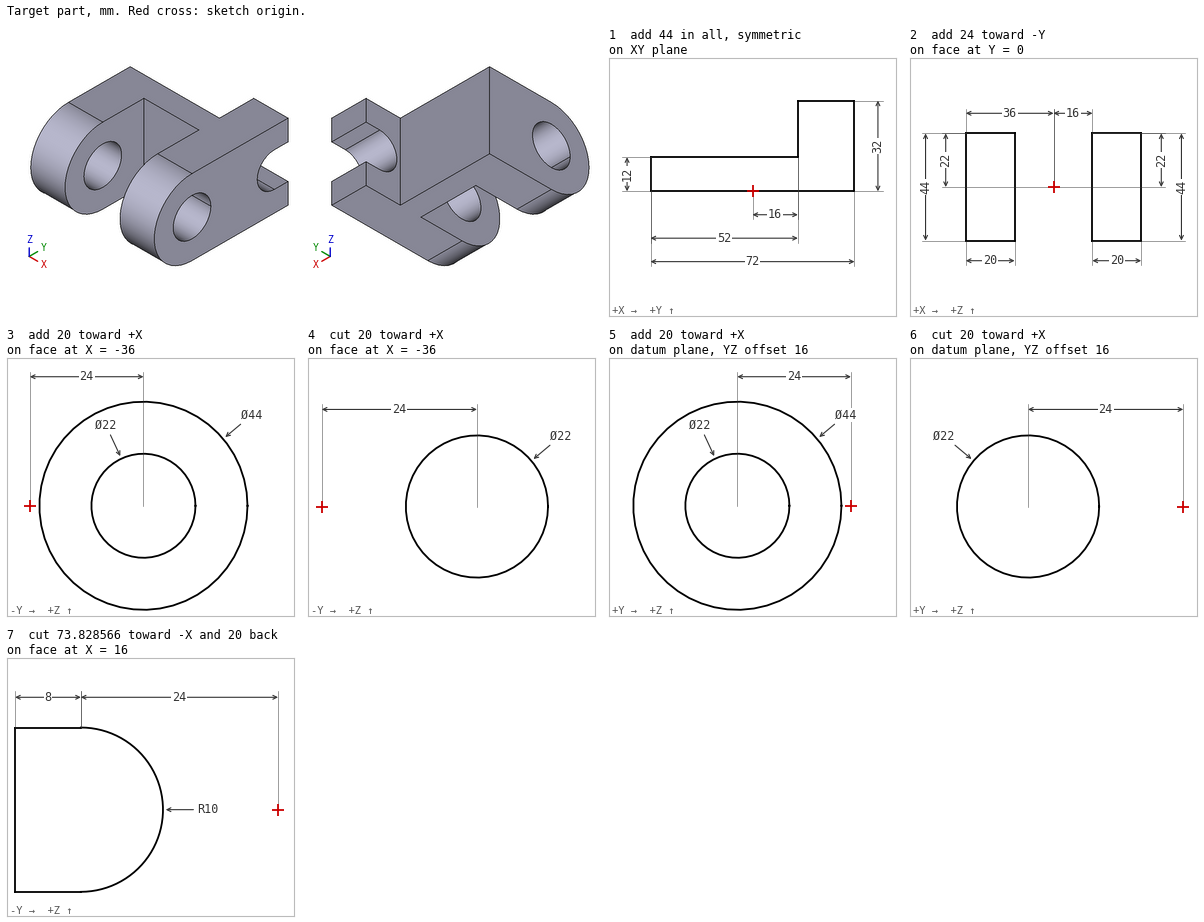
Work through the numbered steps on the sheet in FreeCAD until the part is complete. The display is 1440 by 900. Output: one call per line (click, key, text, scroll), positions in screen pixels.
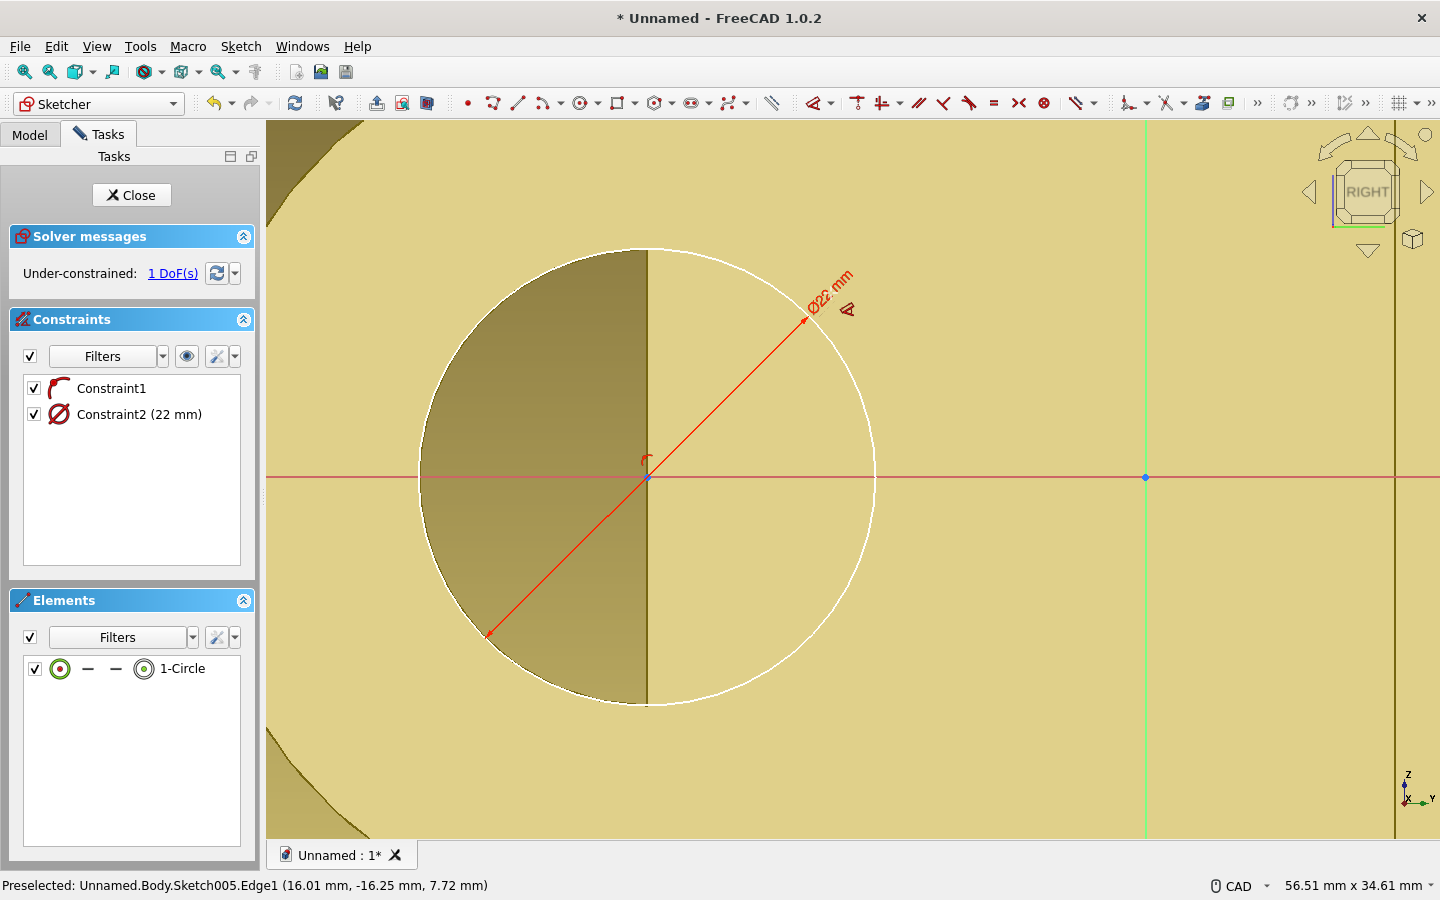
click(647, 477)
click(896, 511)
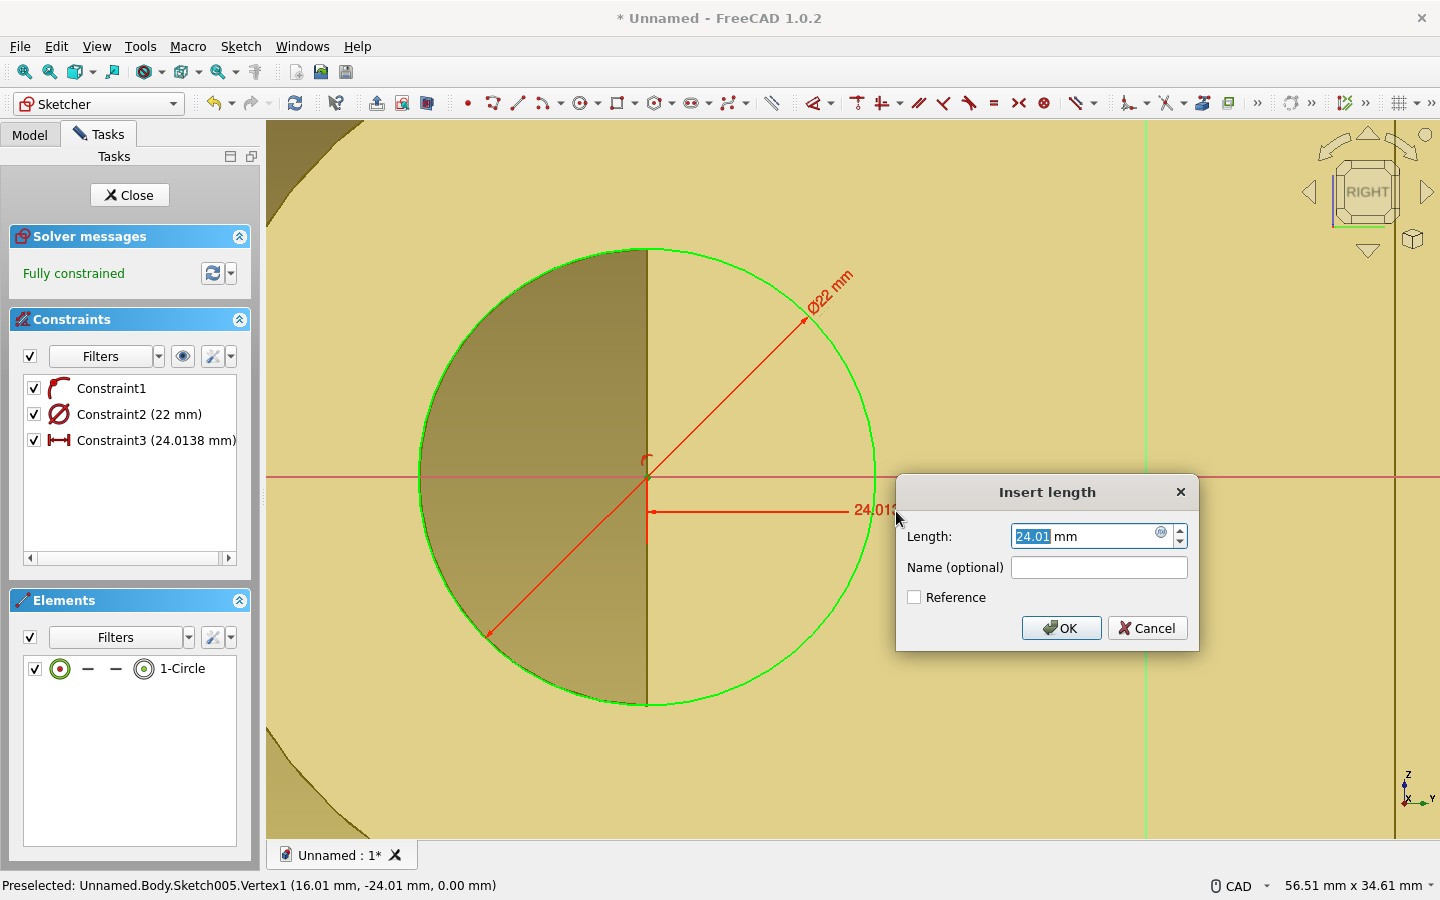
text(24)
key(Return)
key(Escape)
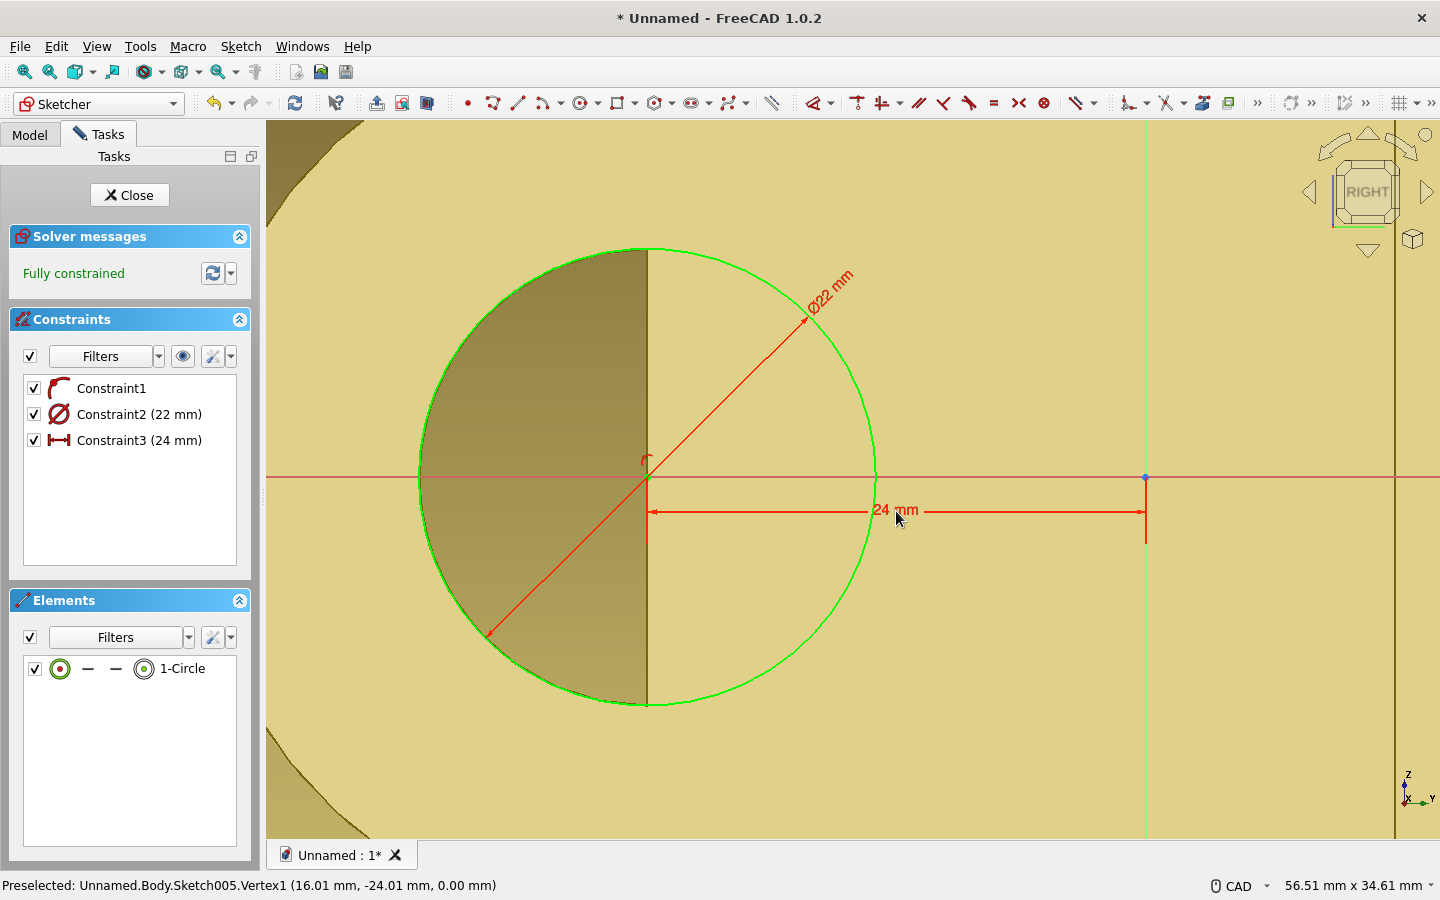
click(130, 195)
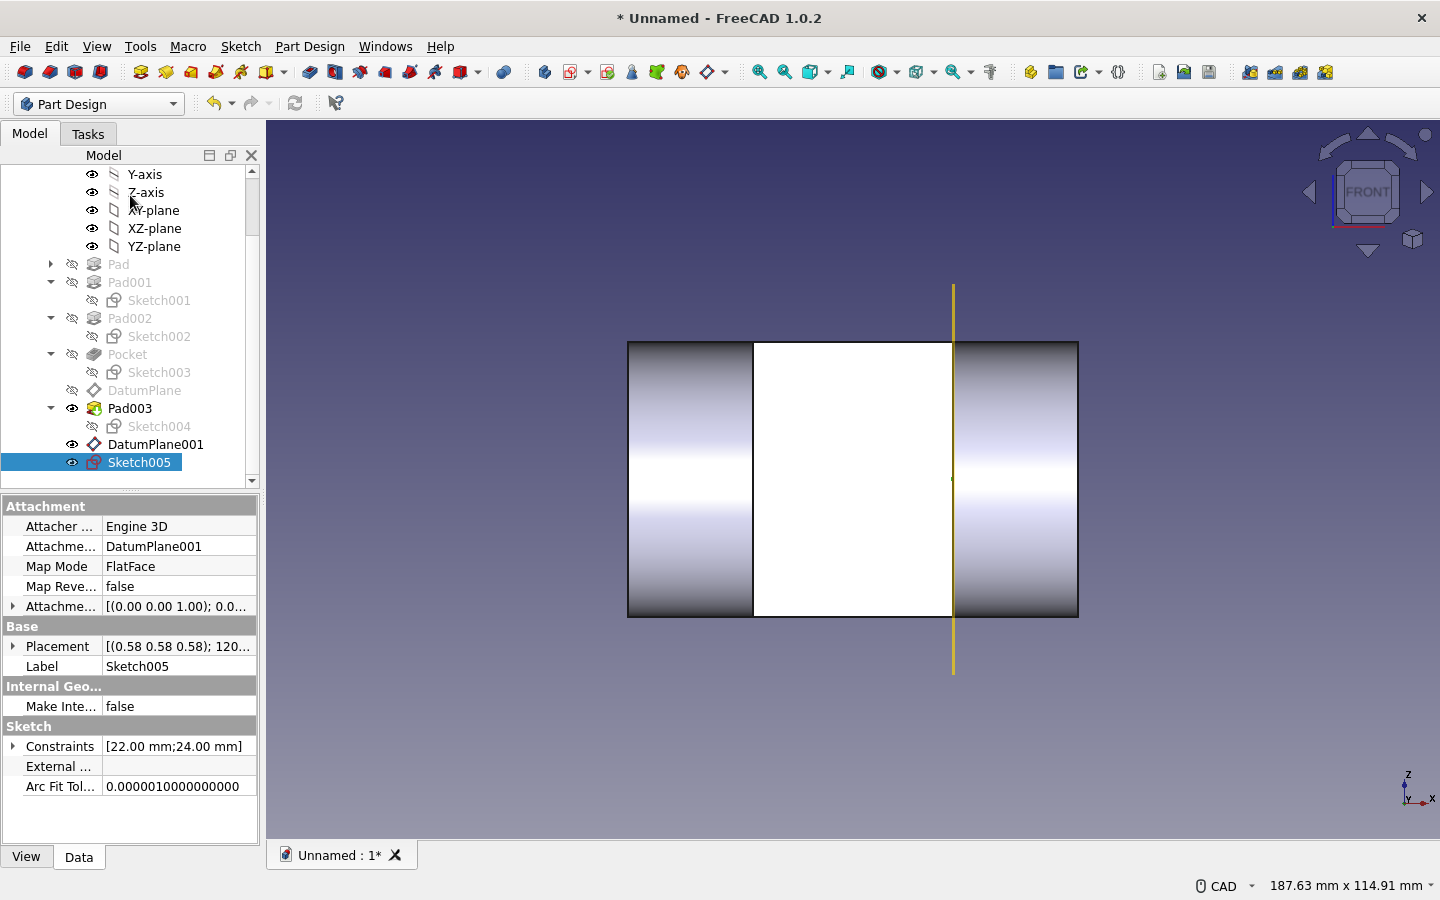
click(310, 72)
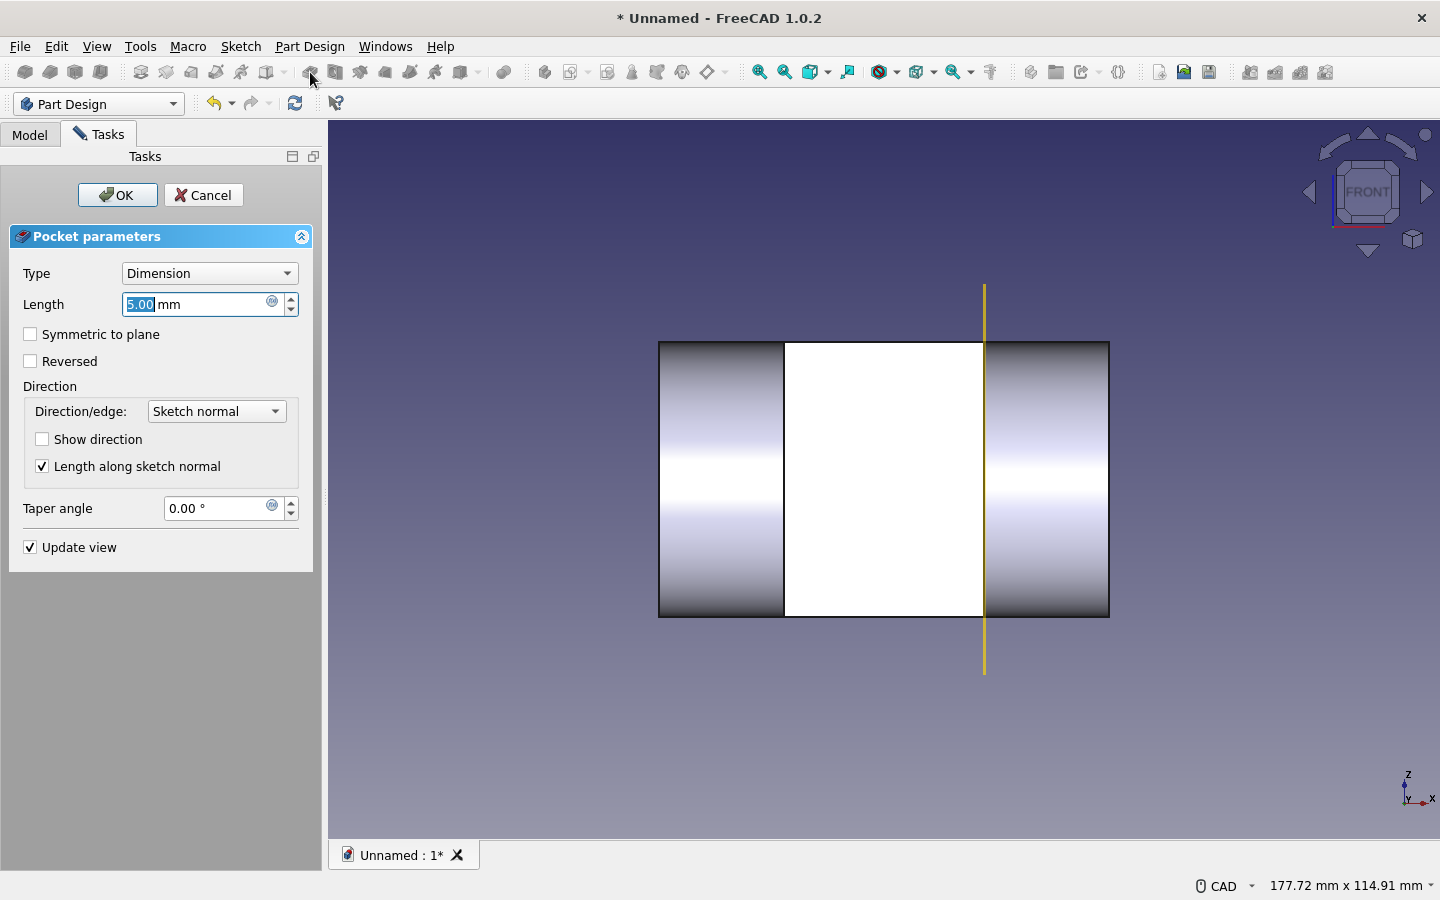
text(20)
key(Tab)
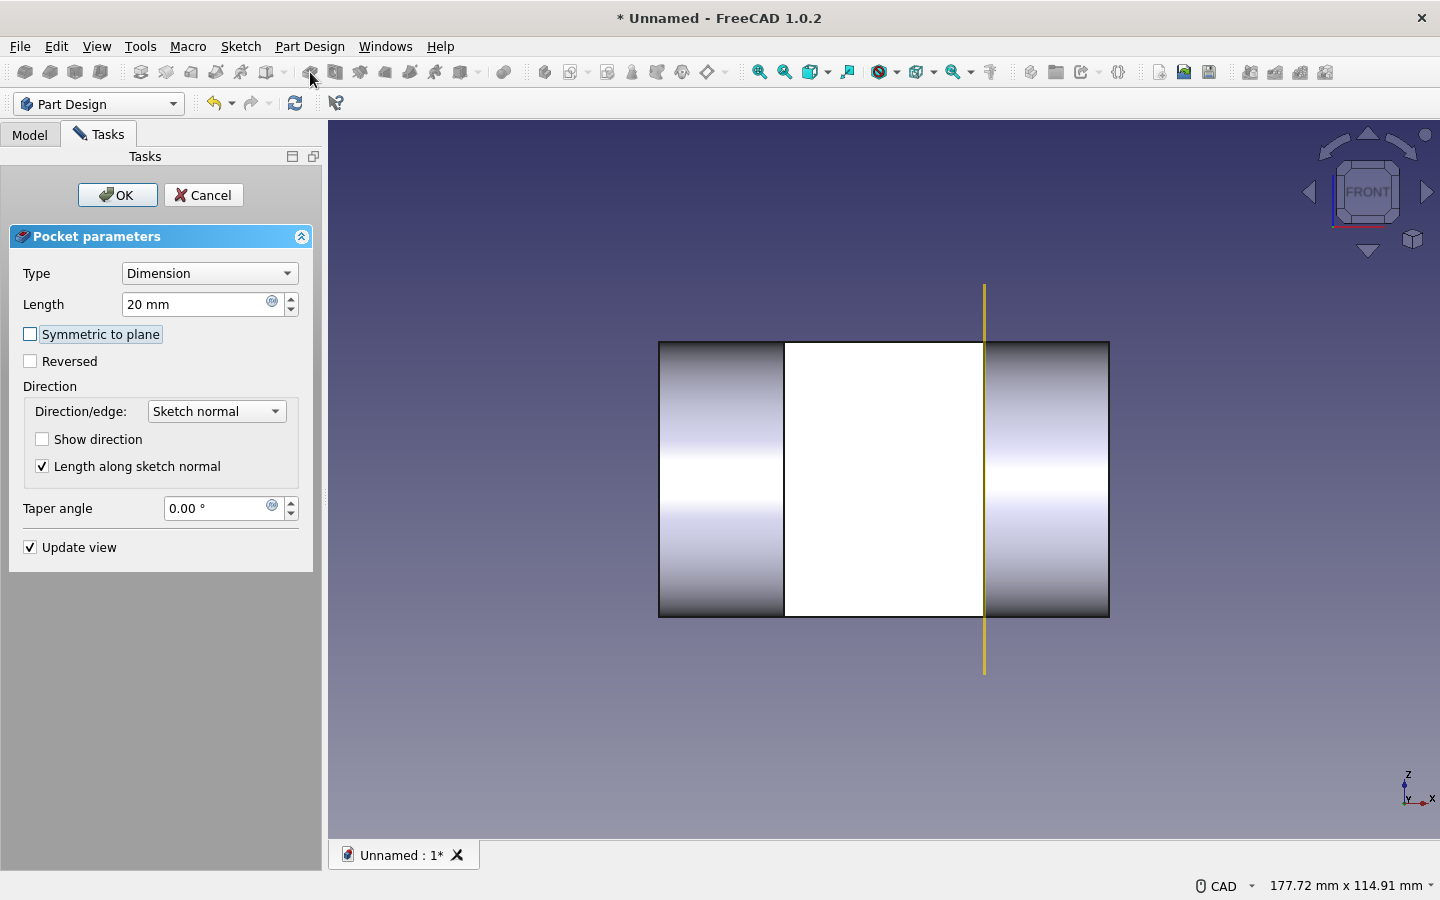
click(31, 361)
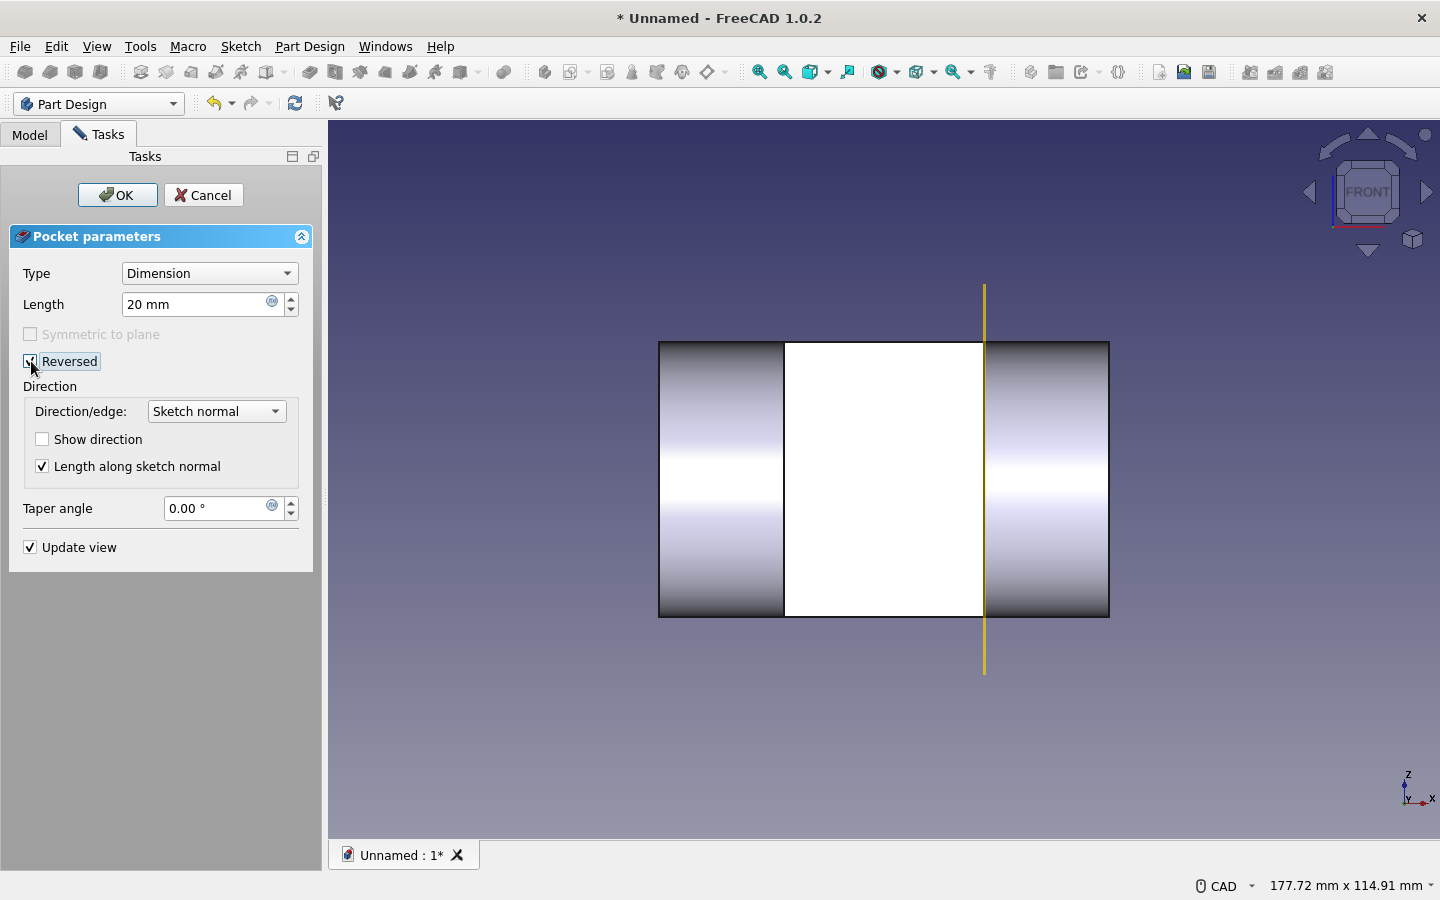
click(118, 195)